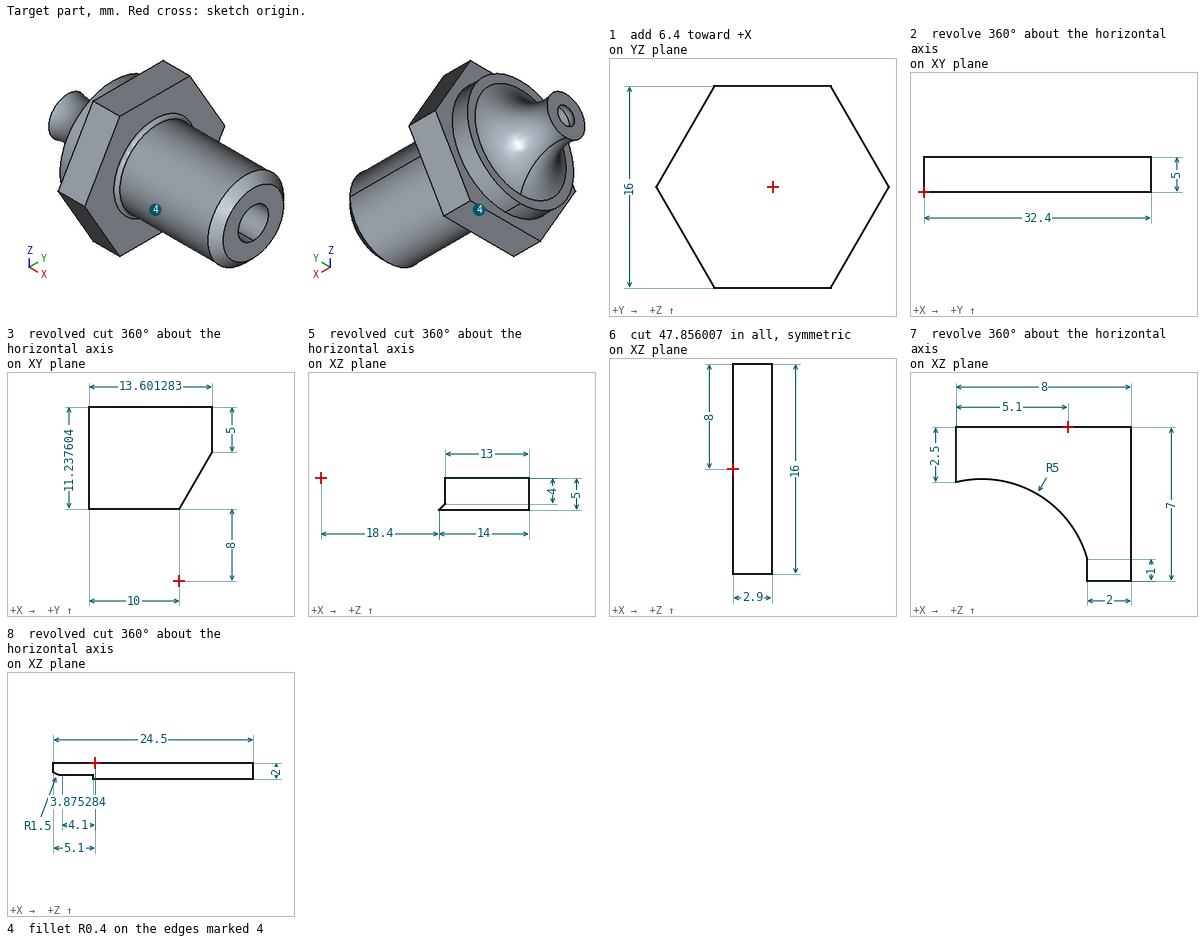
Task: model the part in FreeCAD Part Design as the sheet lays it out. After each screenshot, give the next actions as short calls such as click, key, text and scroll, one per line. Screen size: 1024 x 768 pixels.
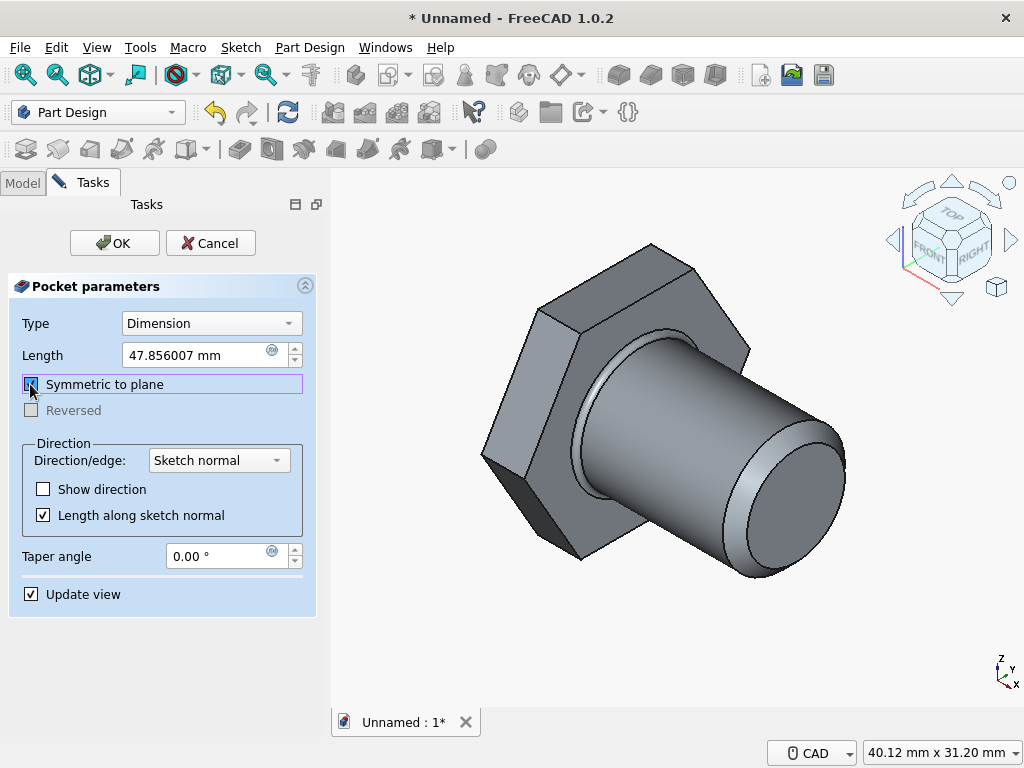
click(115, 243)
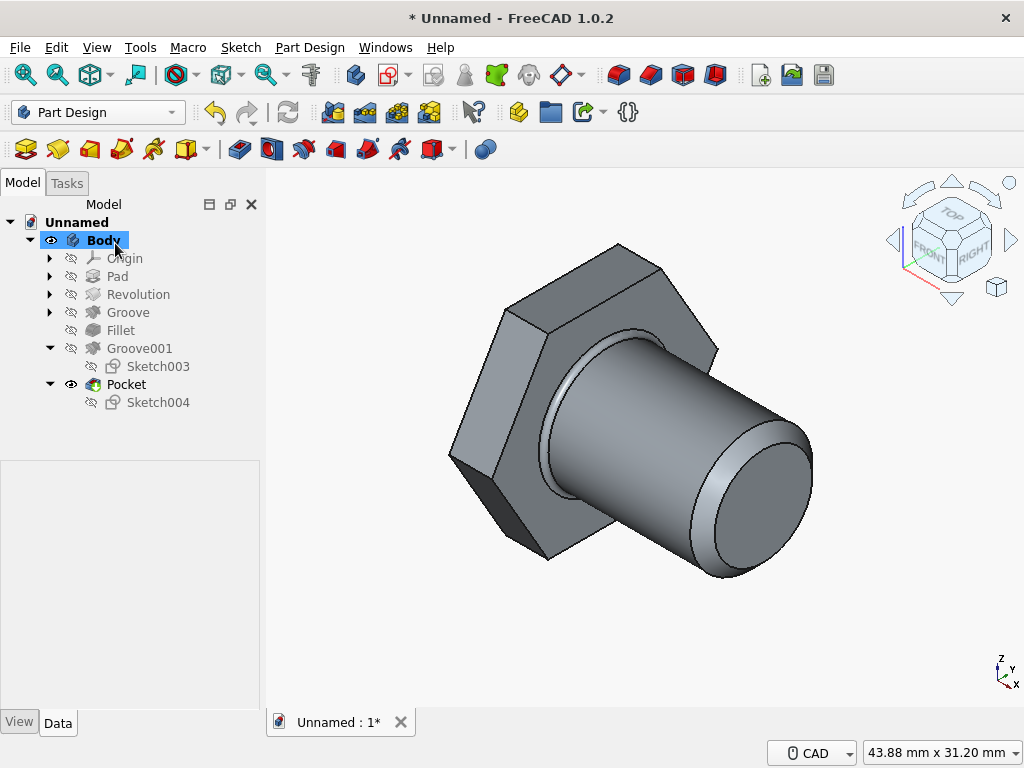
click(388, 76)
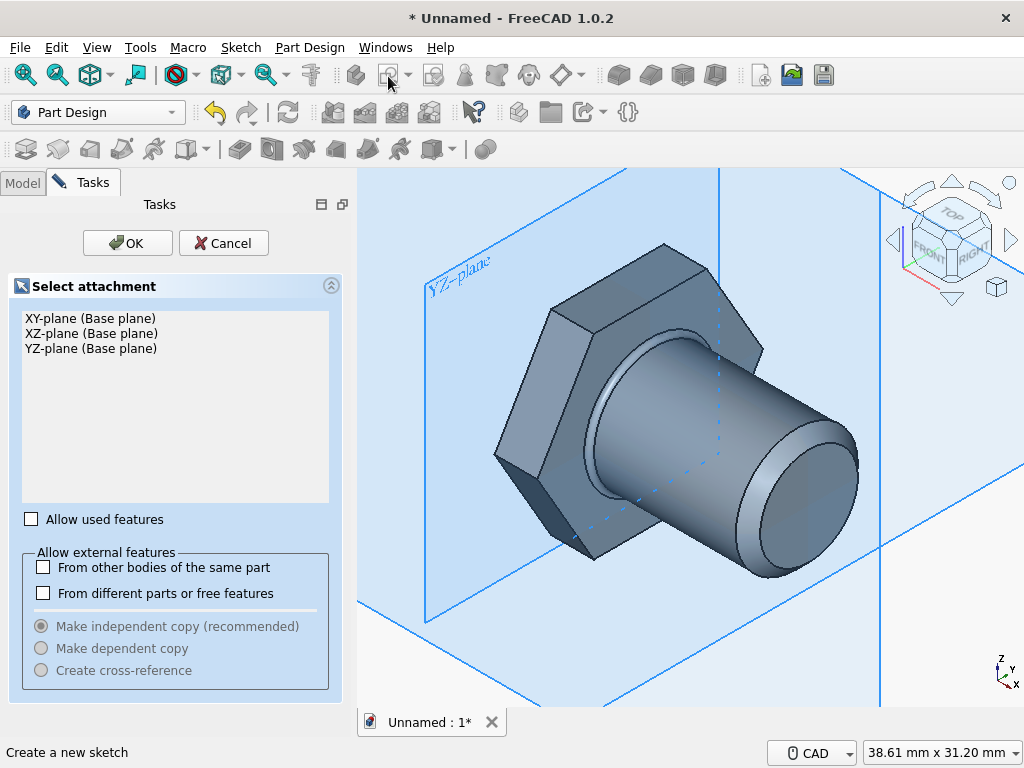
click(82, 334)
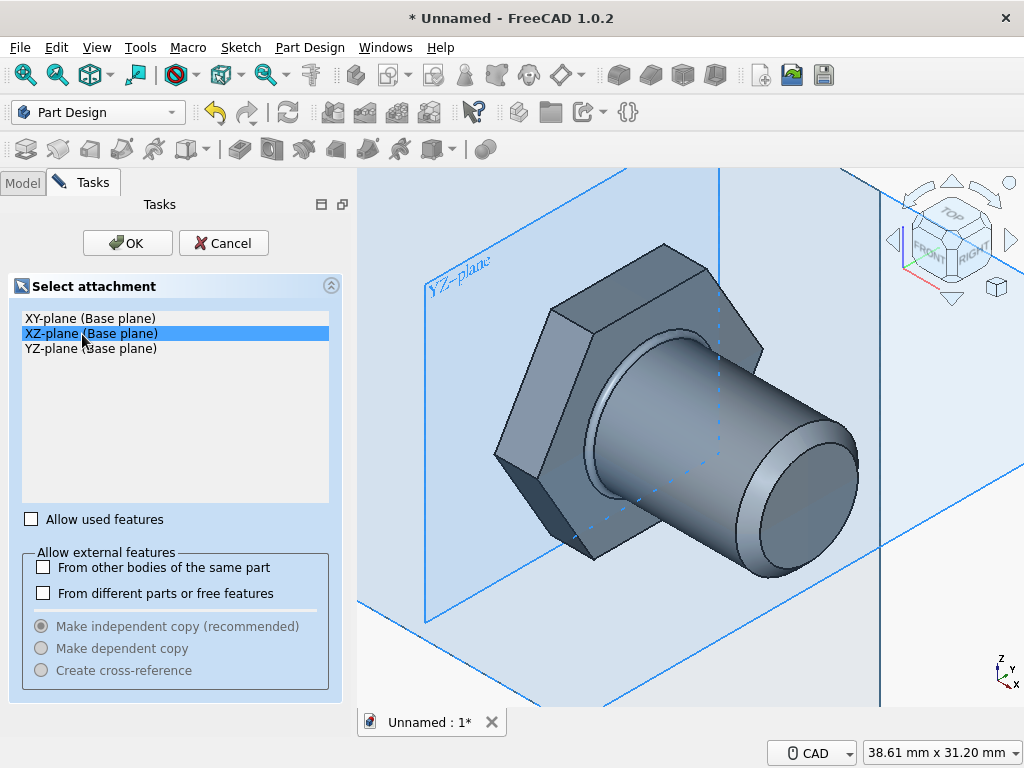
click(128, 243)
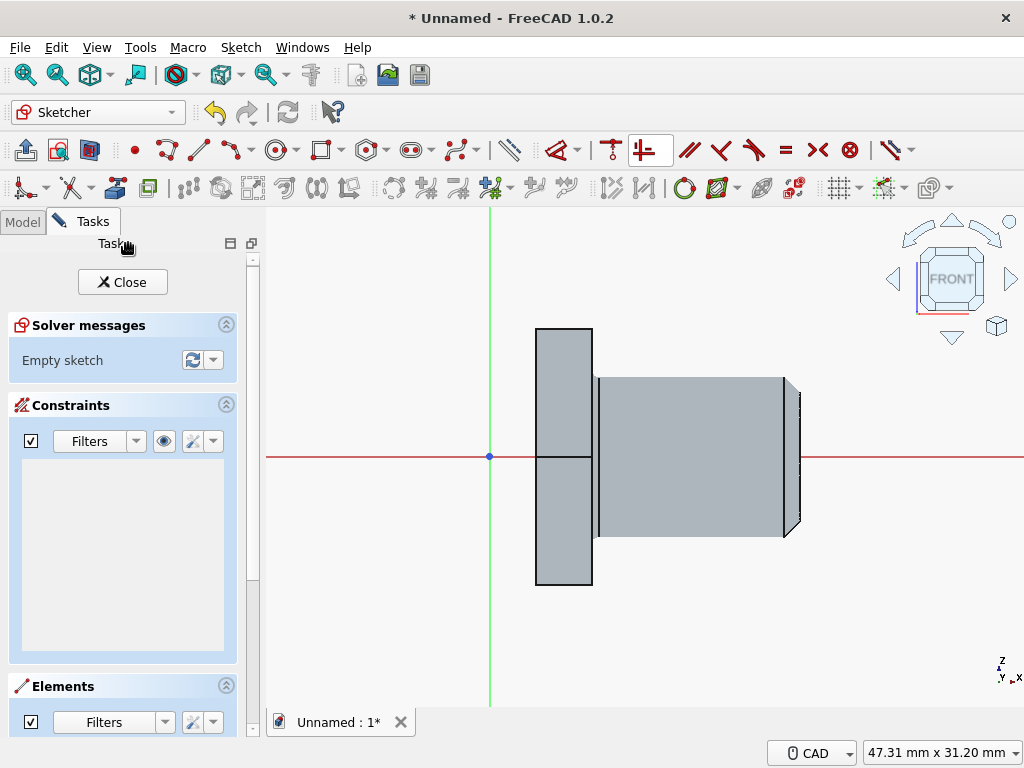
click(90, 150)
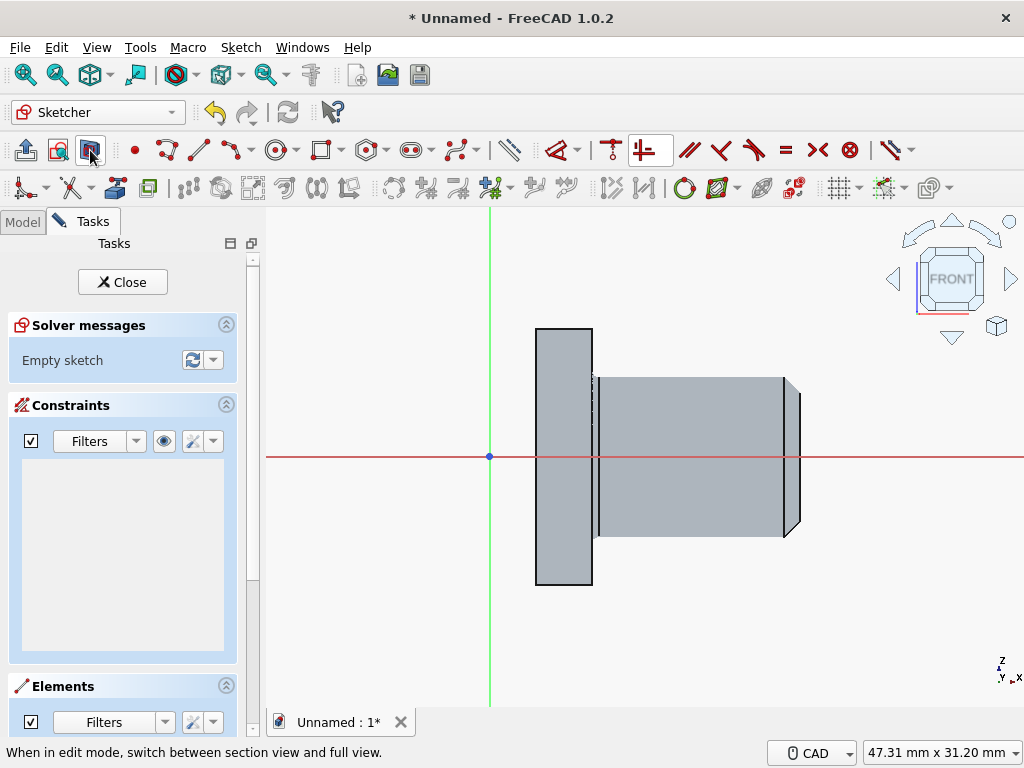
scroll(411, 546, up, 5)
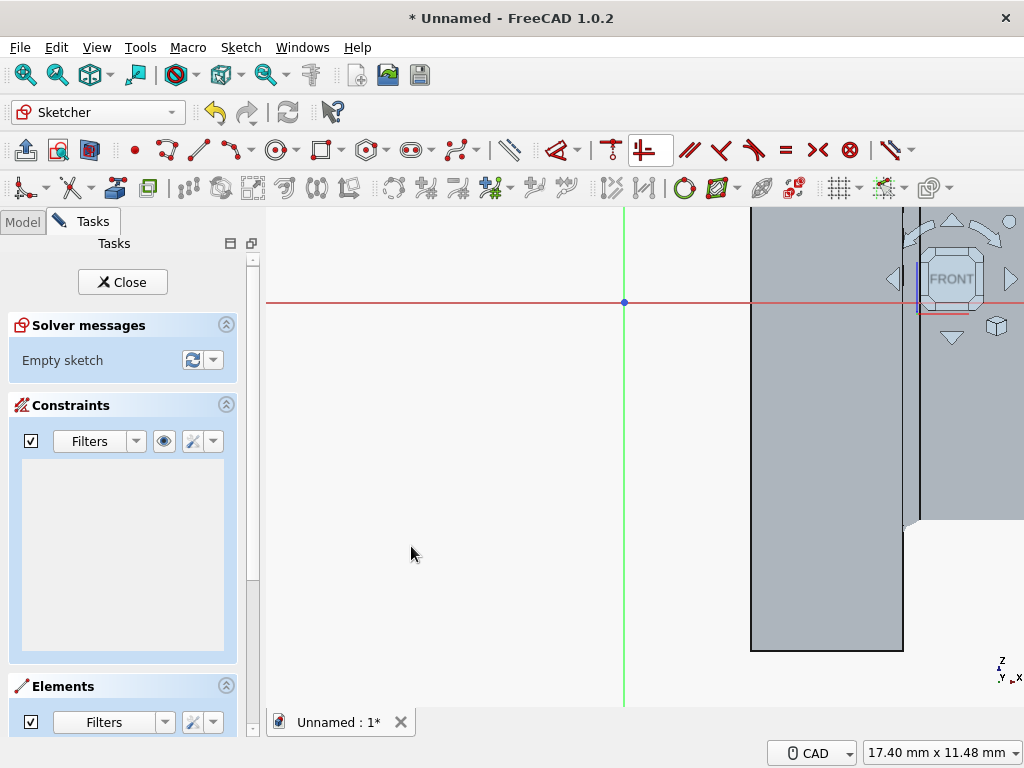
click(168, 150)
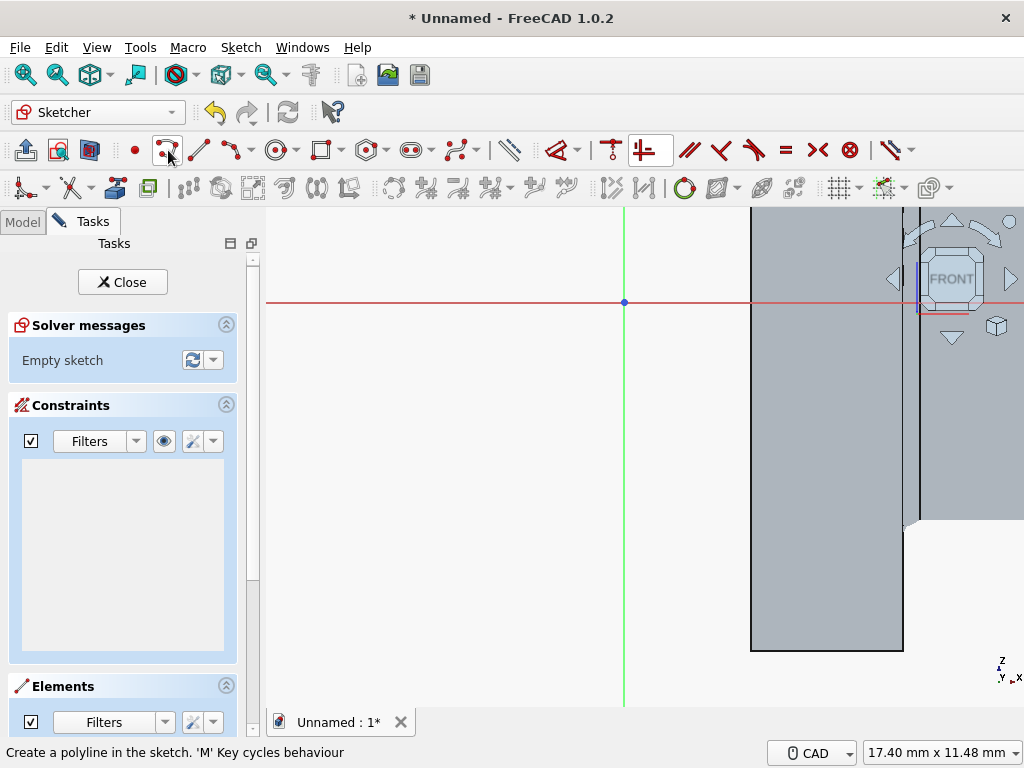
click(402, 412)
click(402, 303)
click(751, 312)
click(751, 608)
click(663, 608)
click(663, 564)
right_click(663, 564)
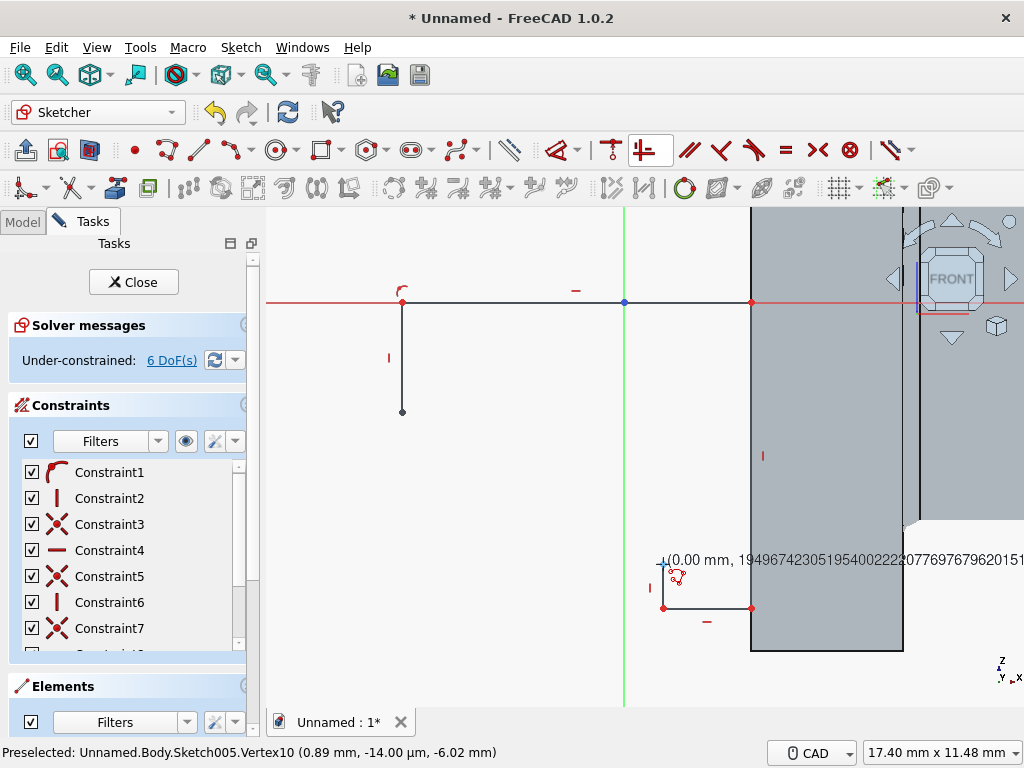
click(232, 150)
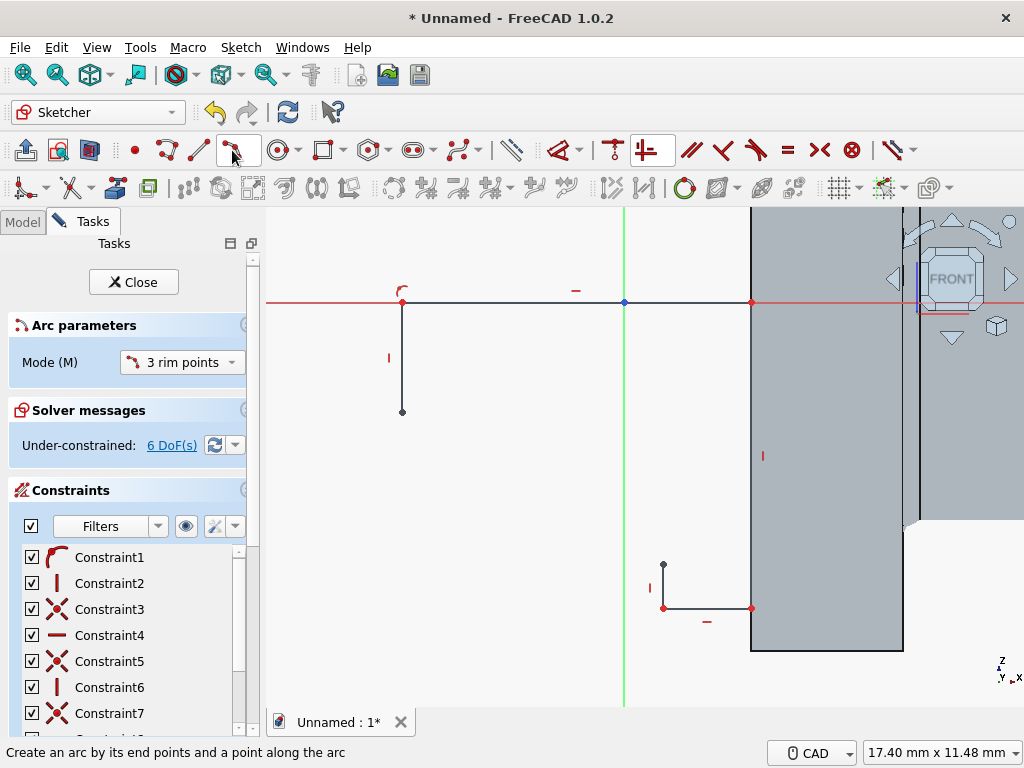
click(663, 565)
click(402, 413)
click(564, 435)
key(Escape)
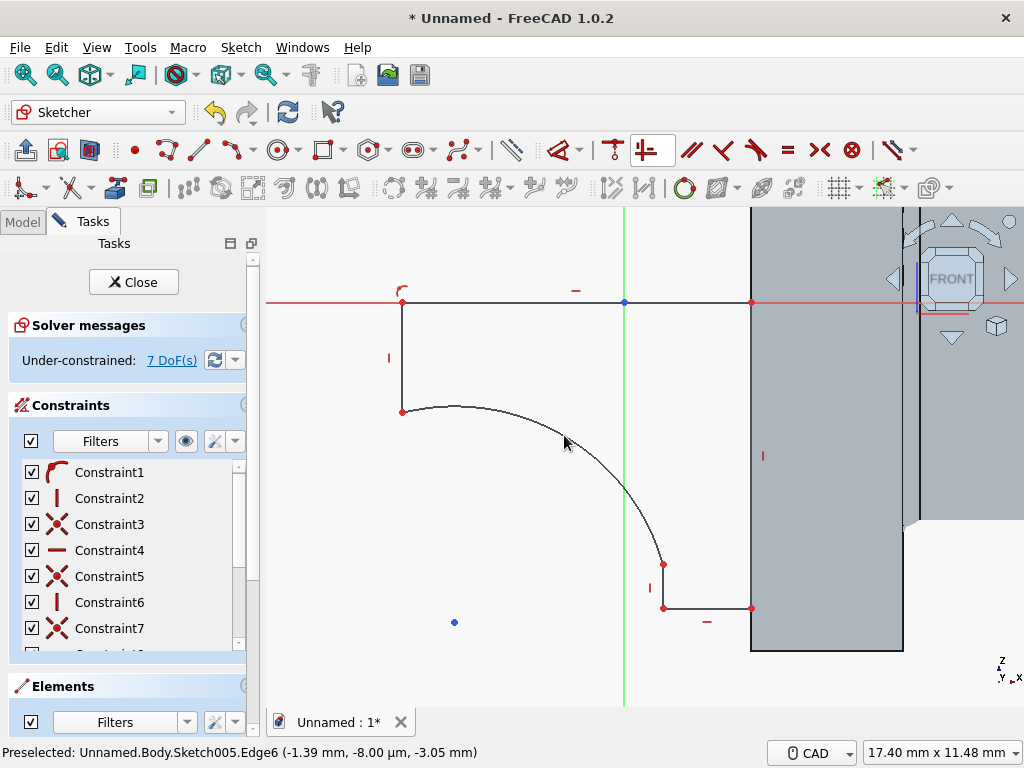
click(558, 150)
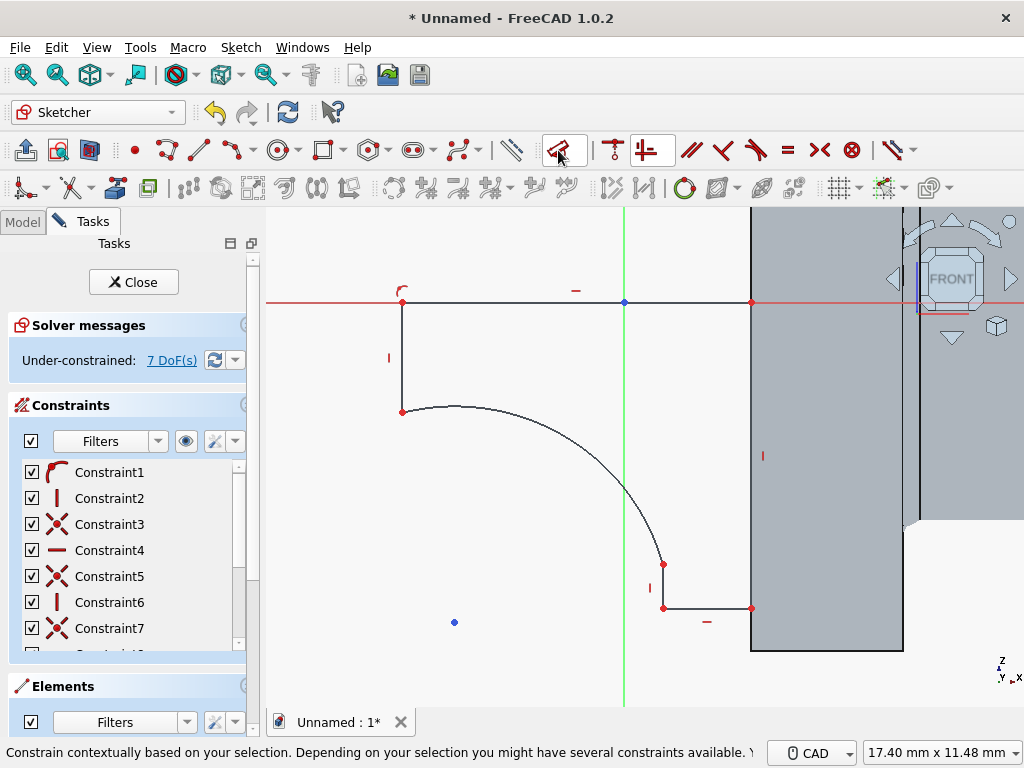
scroll(615, 478, up, 3)